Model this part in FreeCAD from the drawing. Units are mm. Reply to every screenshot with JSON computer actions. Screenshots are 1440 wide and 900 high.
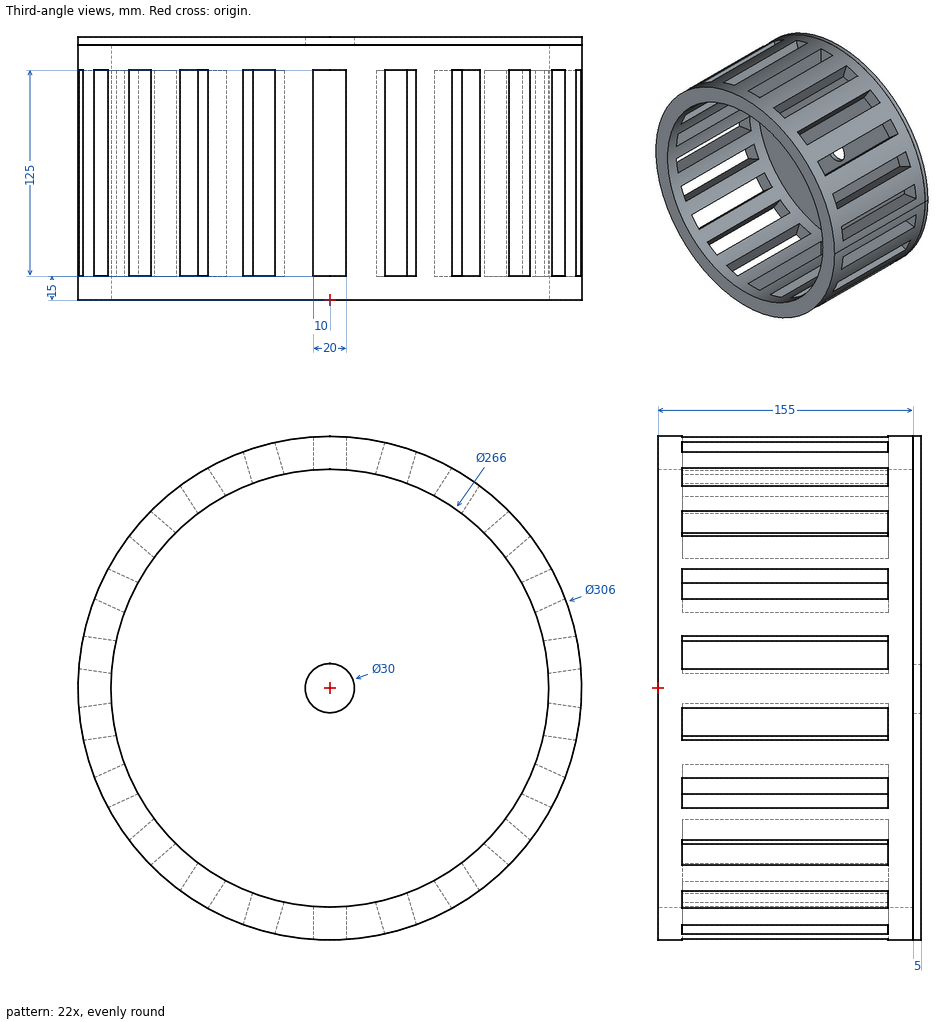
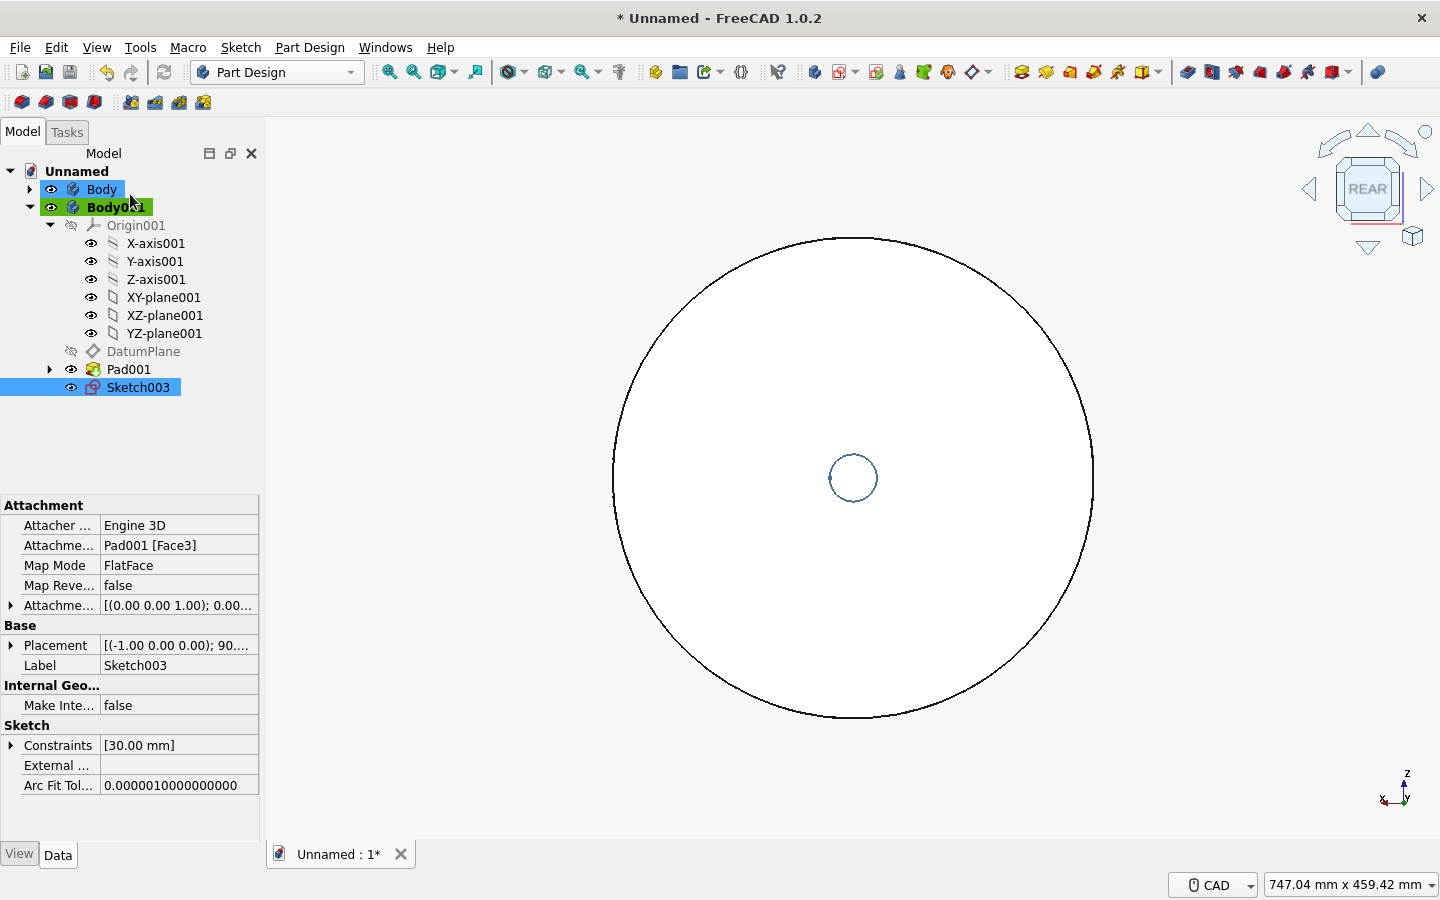
{"action": "left_click", "coordinate": [1188, 72]}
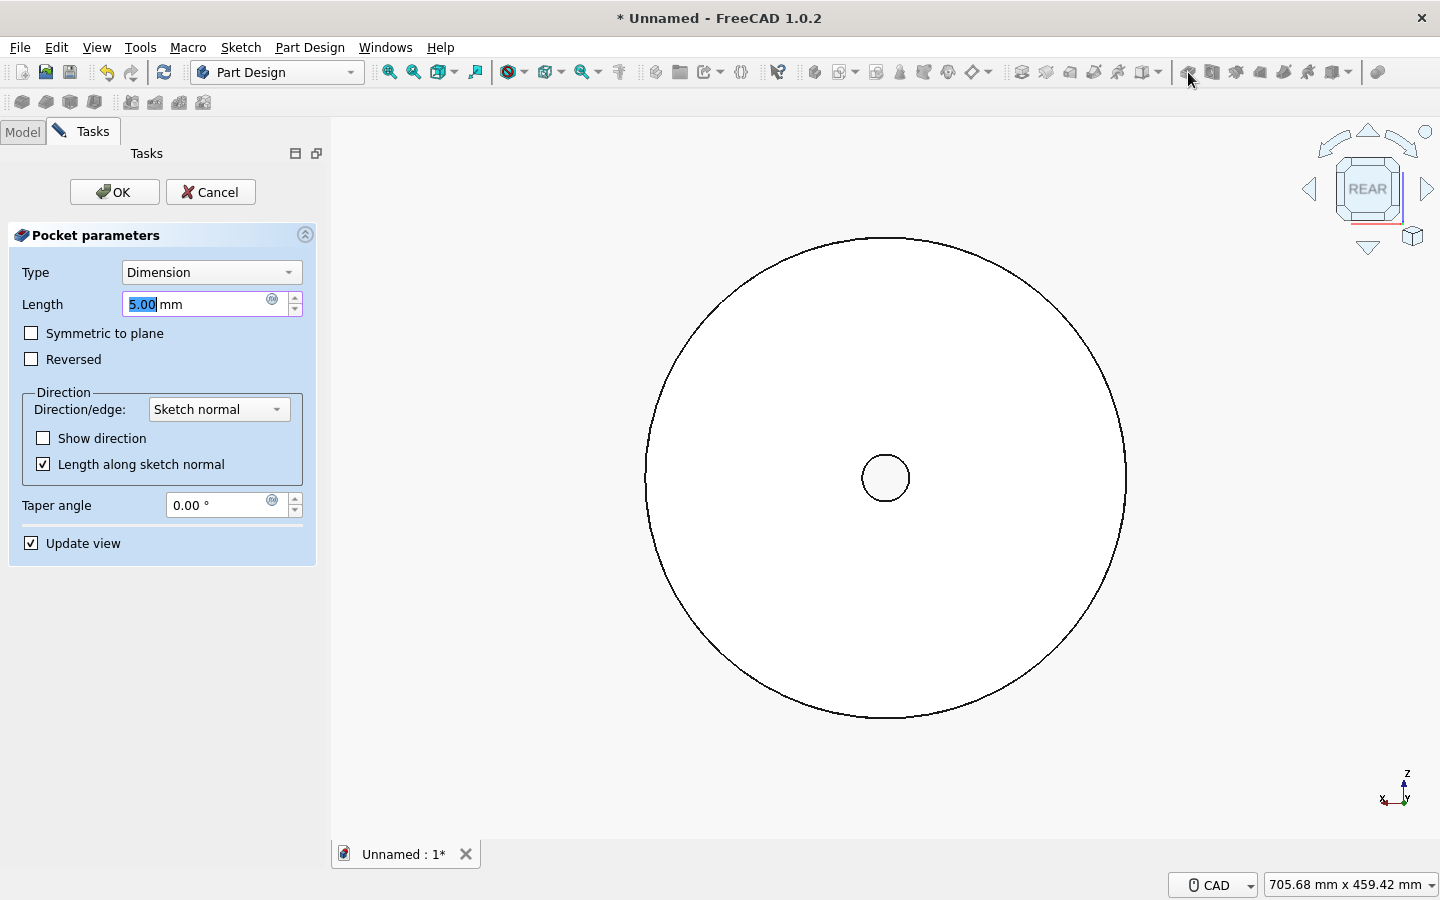
{"action": "left_click", "coordinate": [212, 272]}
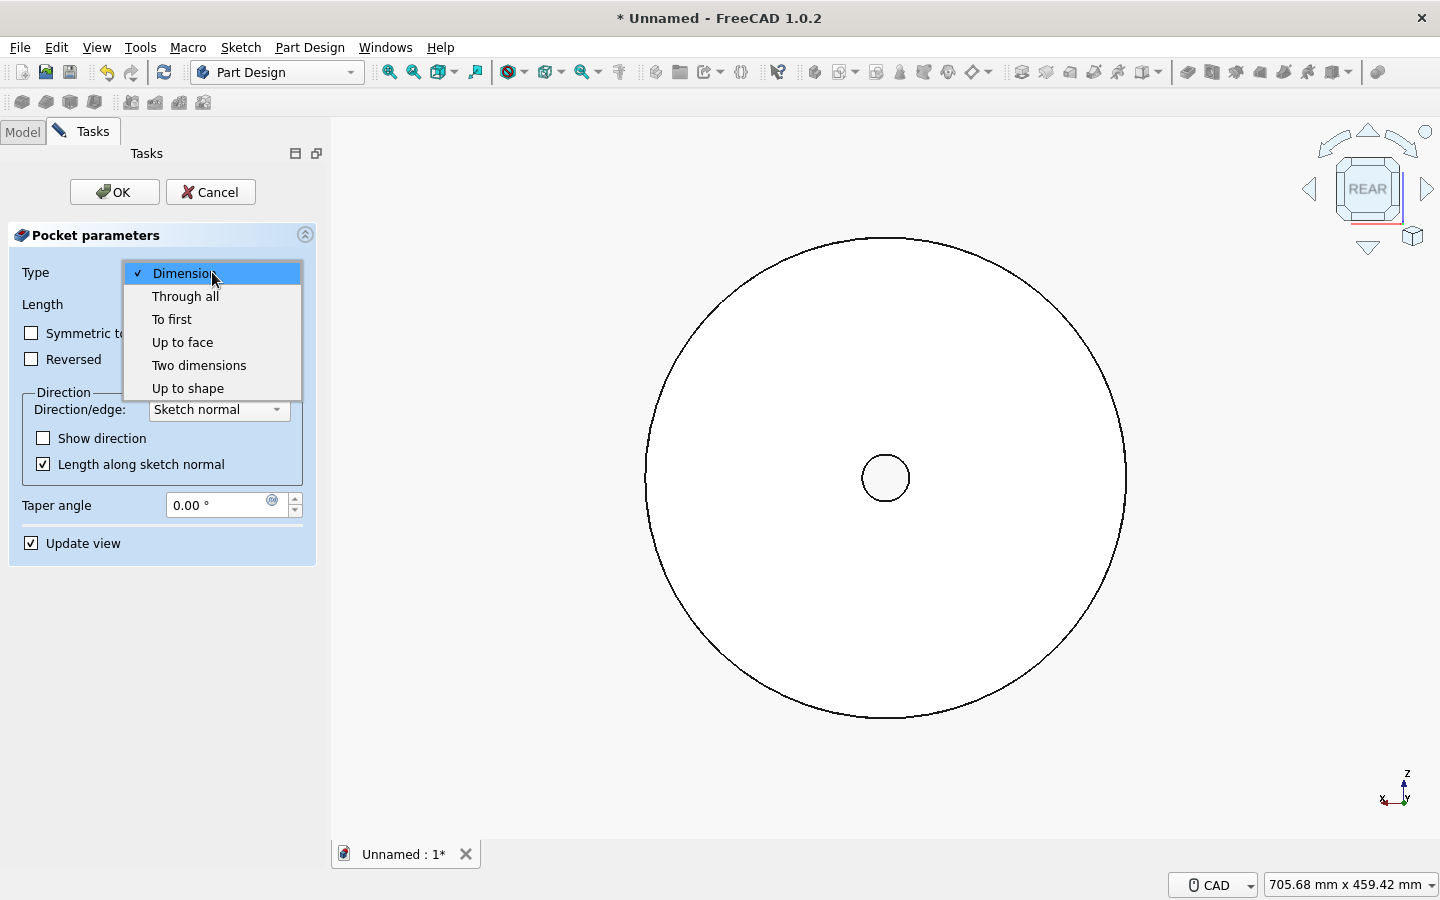
{"action": "left_click", "coordinate": [212, 296]}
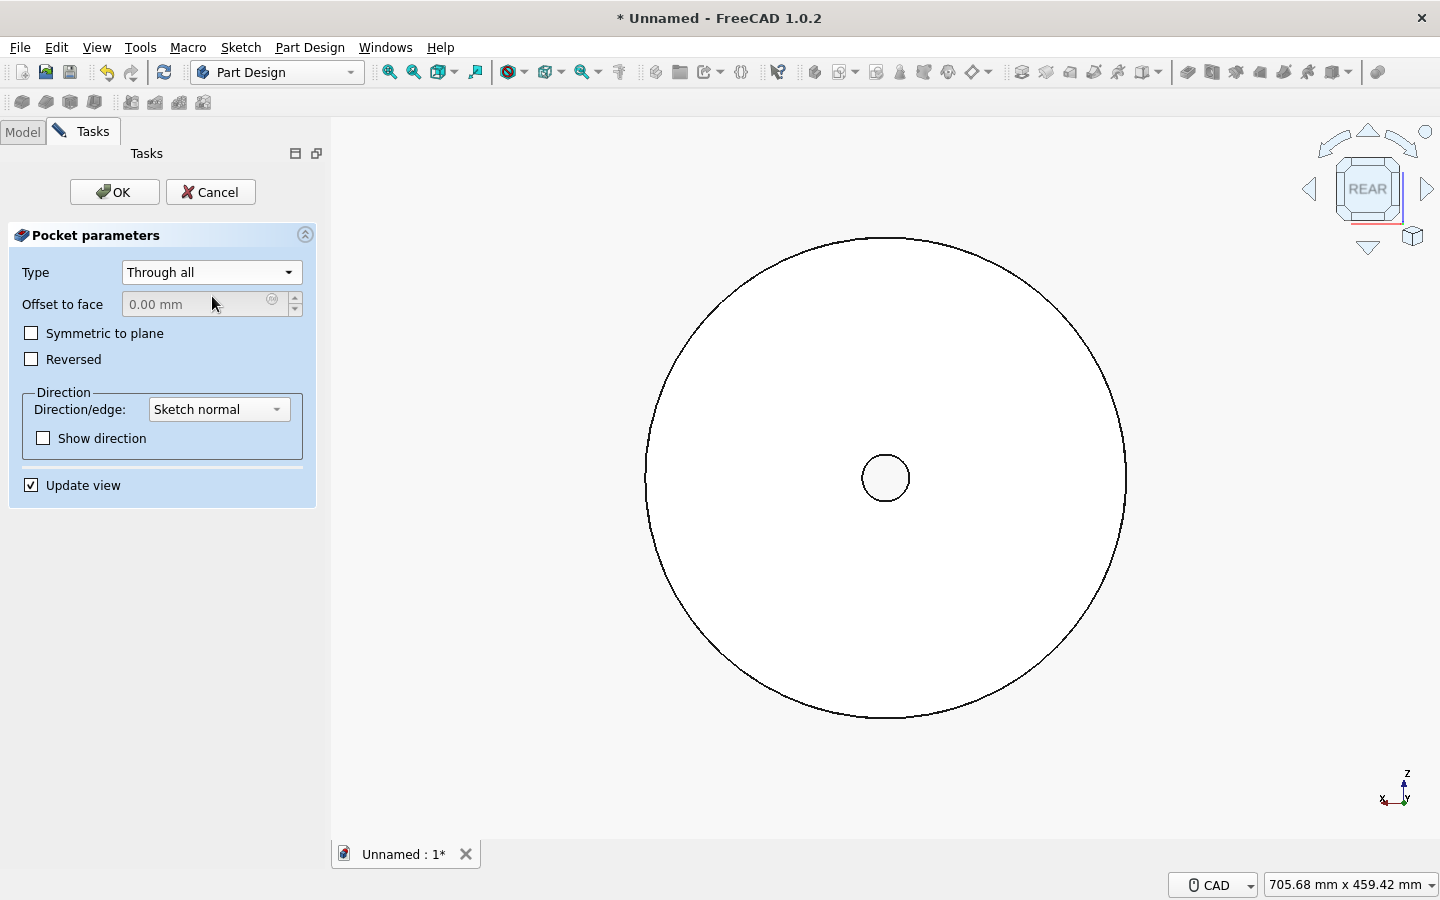
{"action": "left_click", "coordinate": [115, 192]}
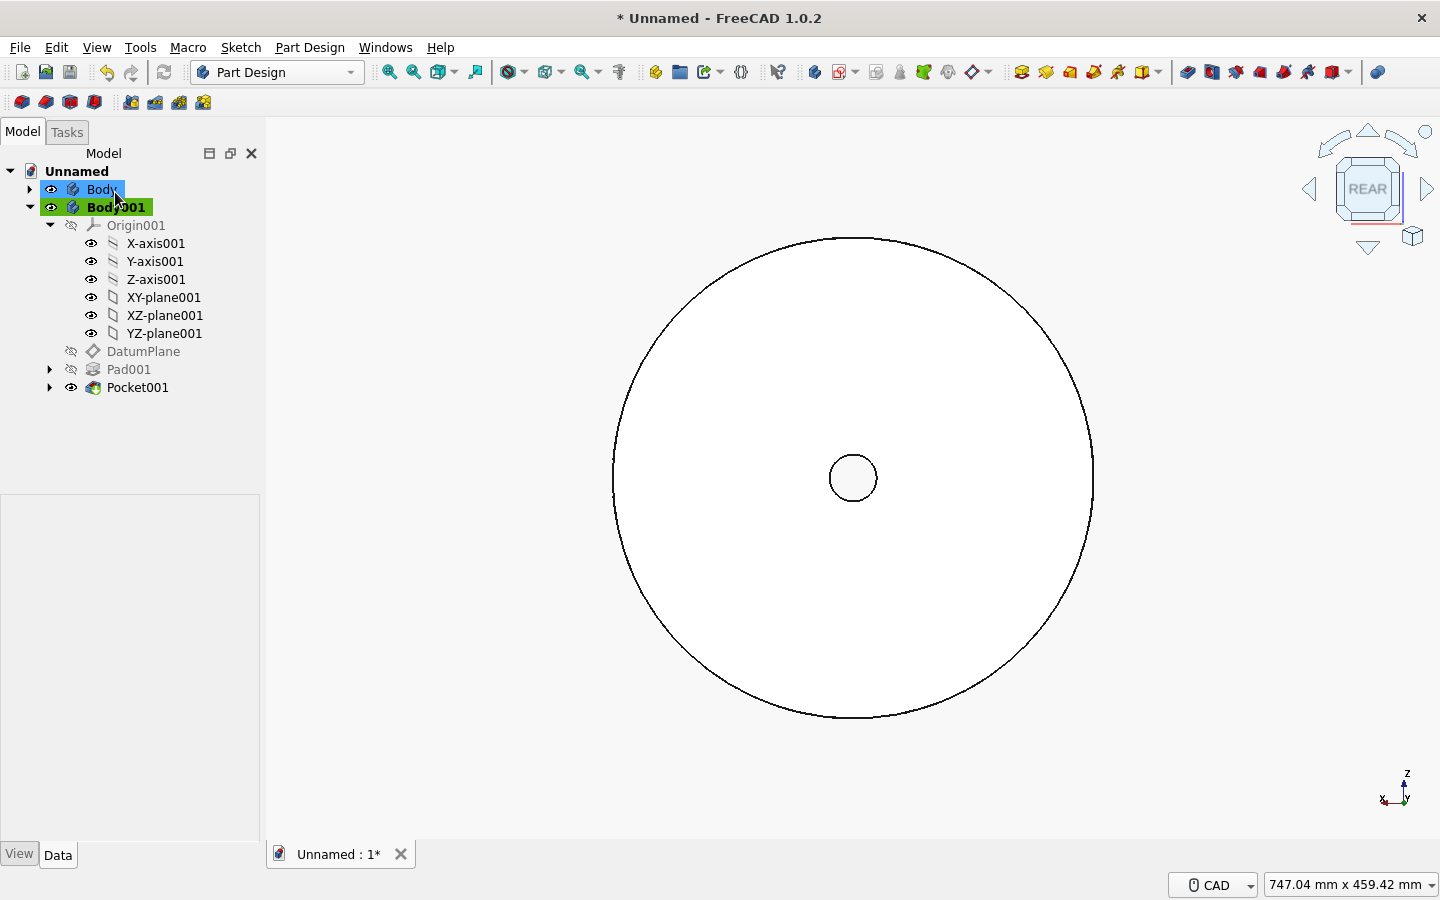
{"action": "key", "text": "0"}